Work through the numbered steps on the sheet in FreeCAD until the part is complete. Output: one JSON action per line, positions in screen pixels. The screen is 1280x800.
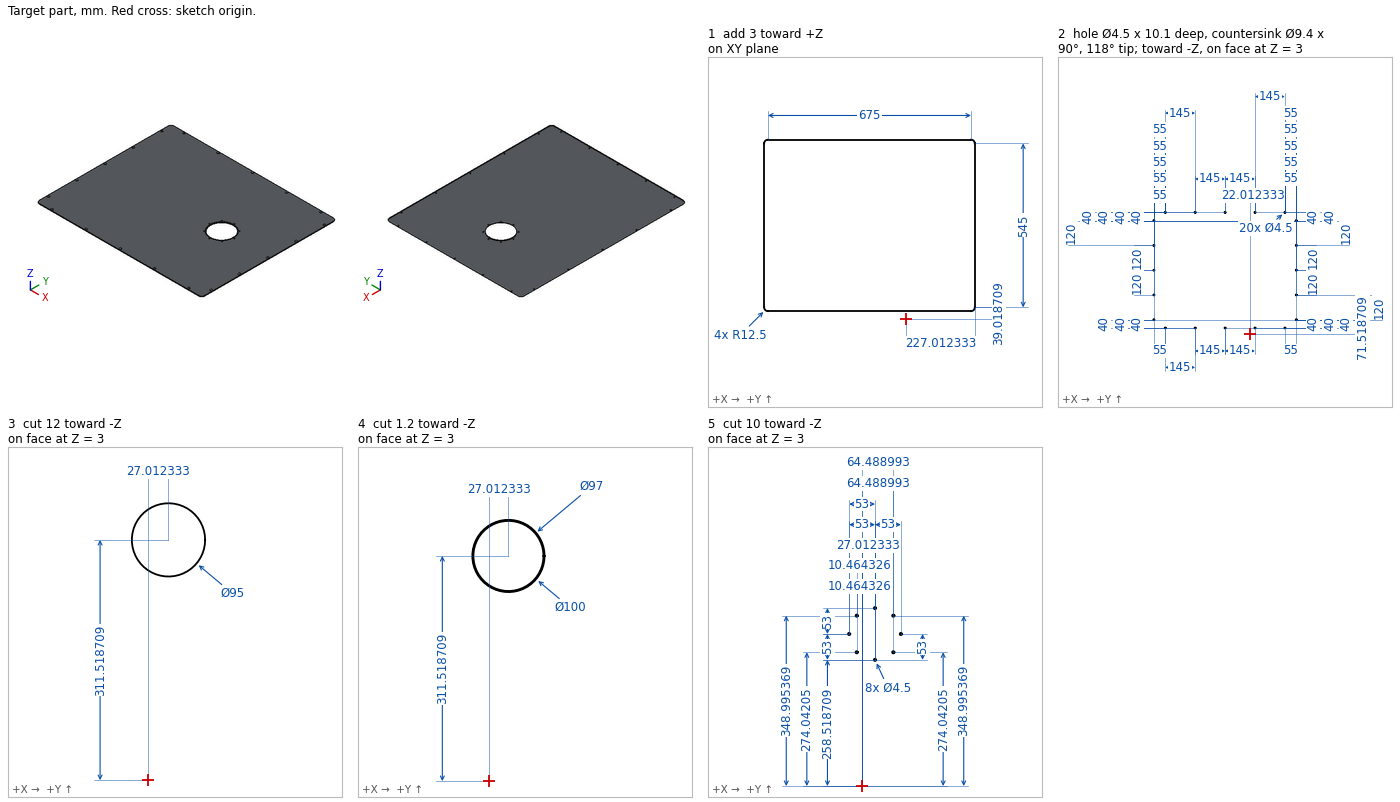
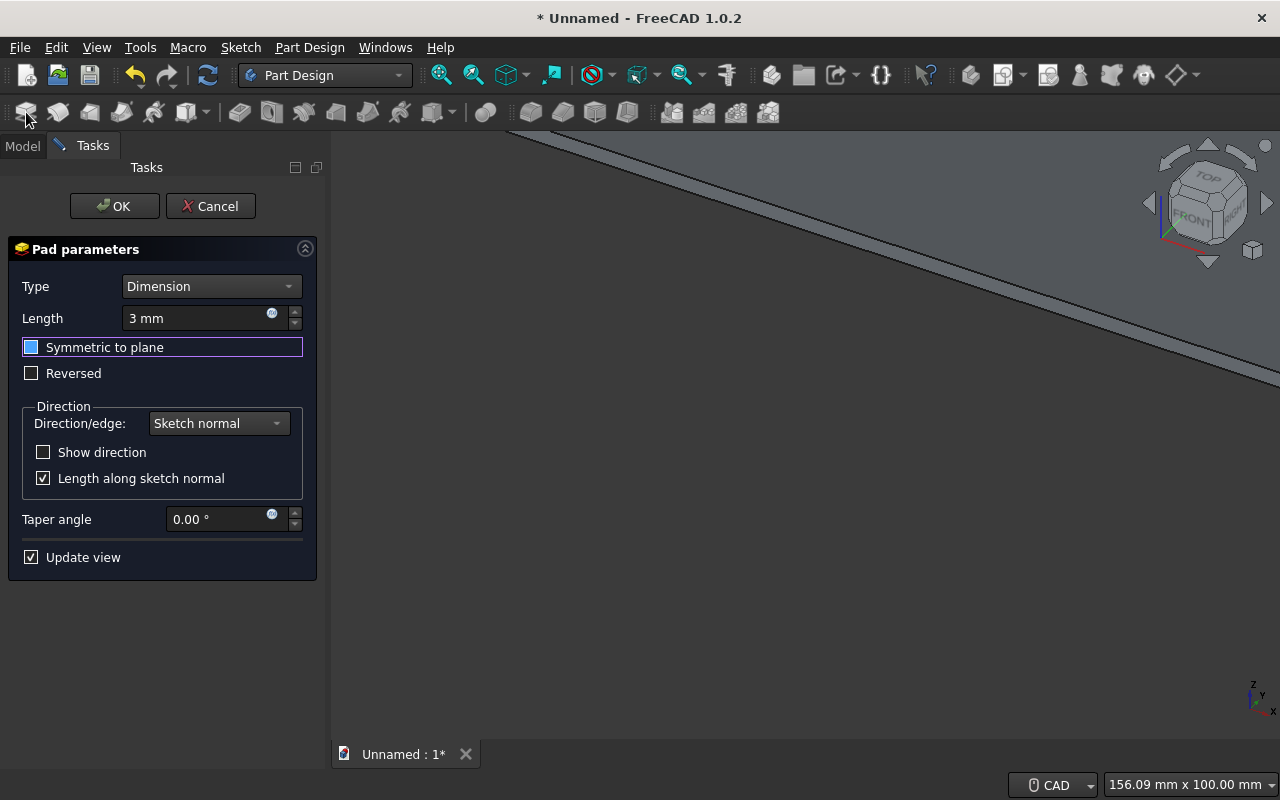
{"action": "left_click", "coordinate": [115, 206]}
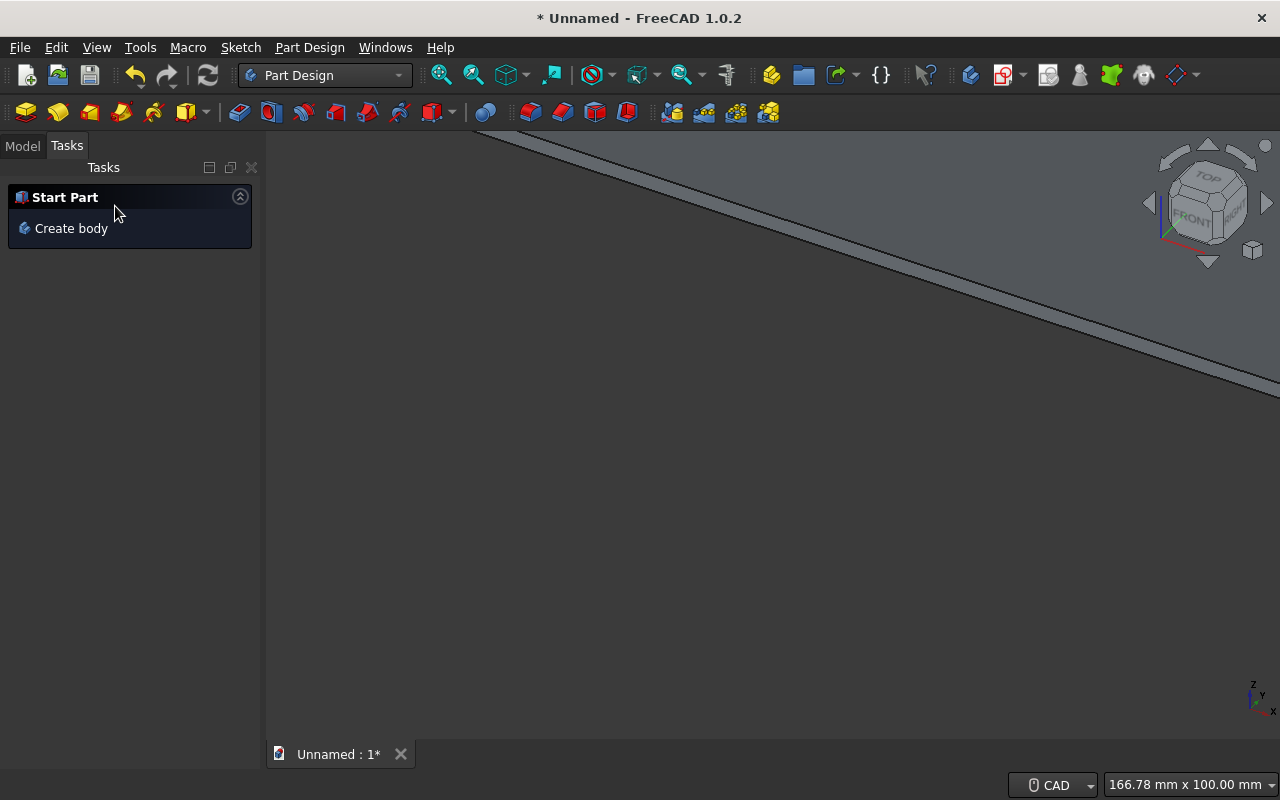
{"action": "left_click", "coordinate": [442, 76]}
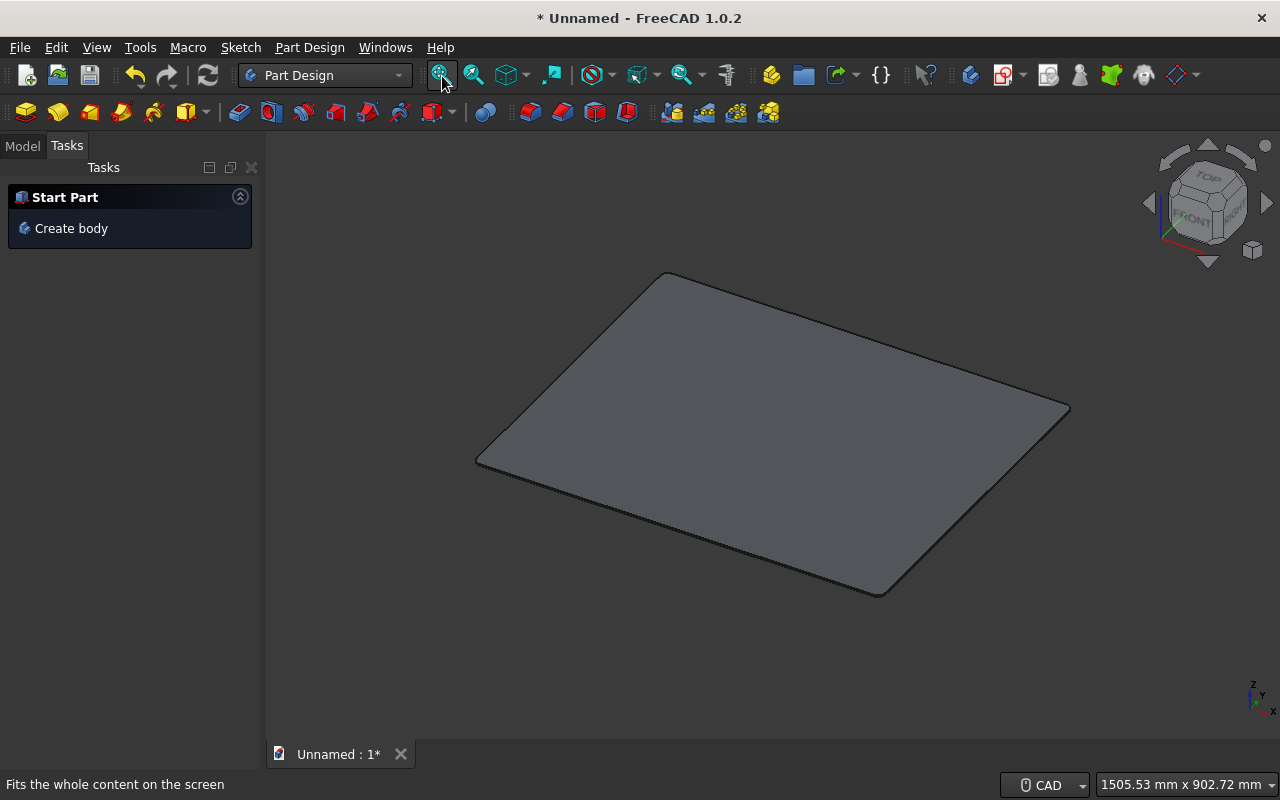
{"action": "left_click", "coordinate": [773, 433]}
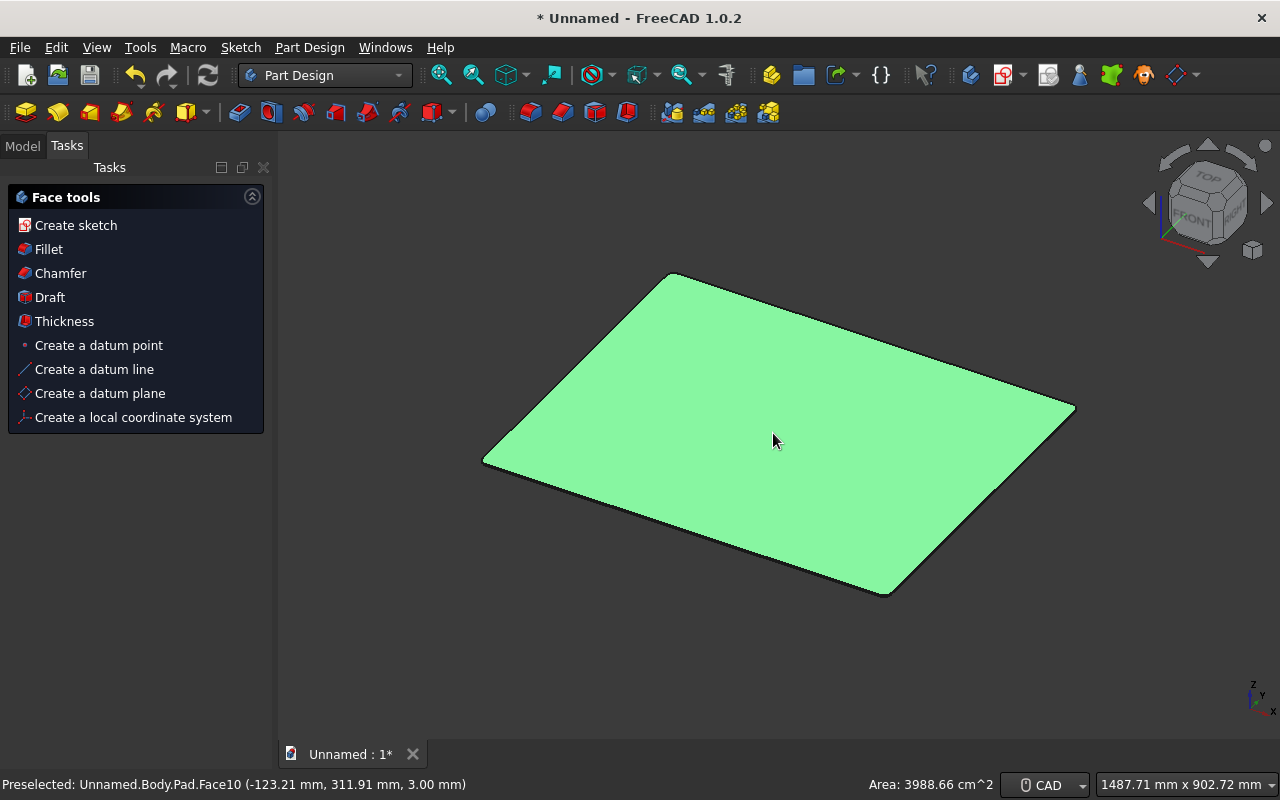
{"action": "left_click", "coordinate": [1004, 76]}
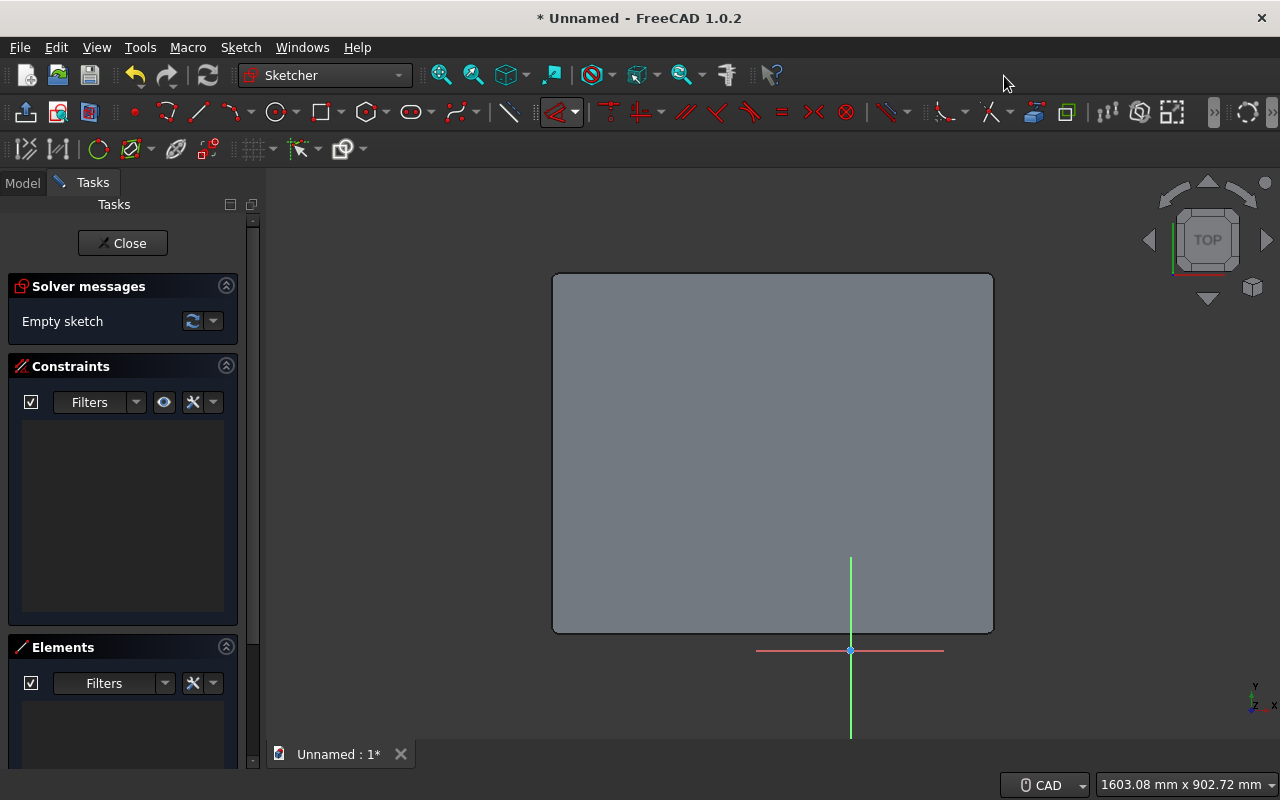
{"action": "left_click", "coordinate": [276, 112]}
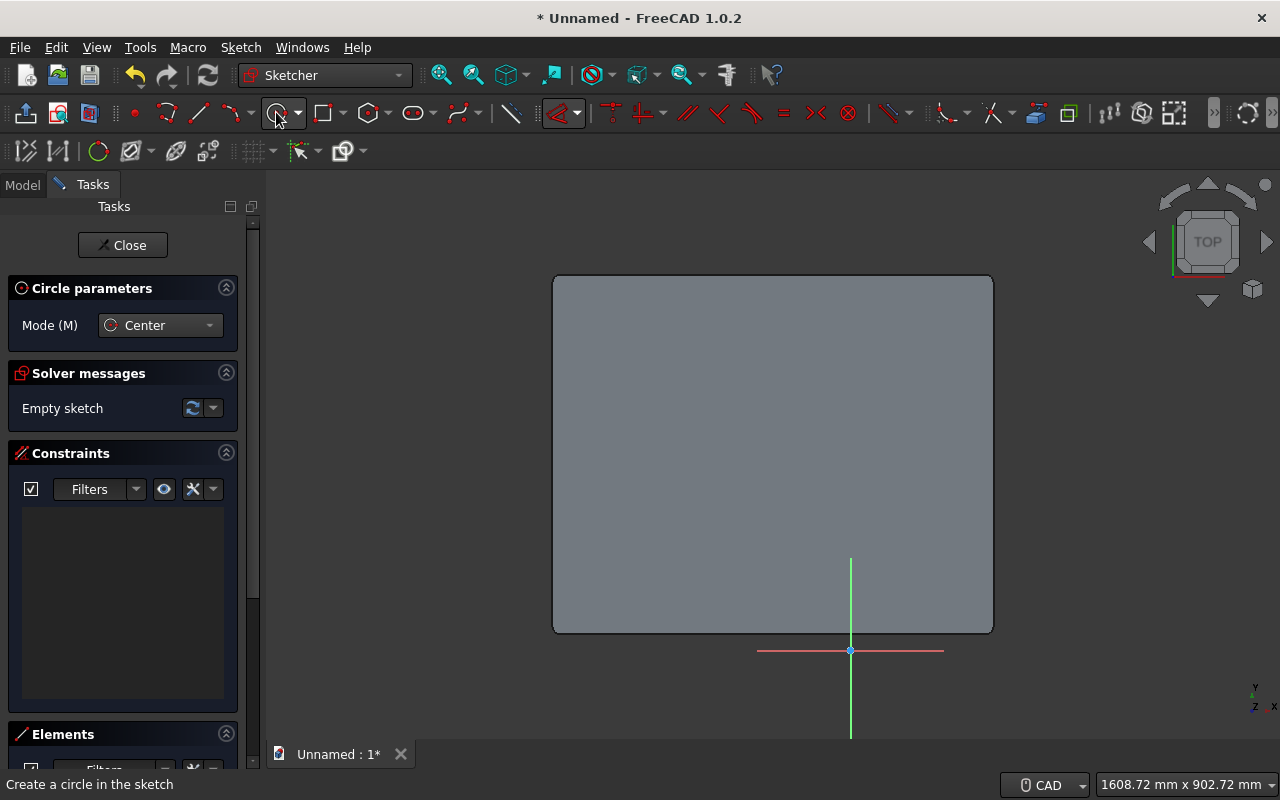
{"action": "scroll", "coordinate": [990, 606], "scroll_direction": "up", "scroll_amount": 14}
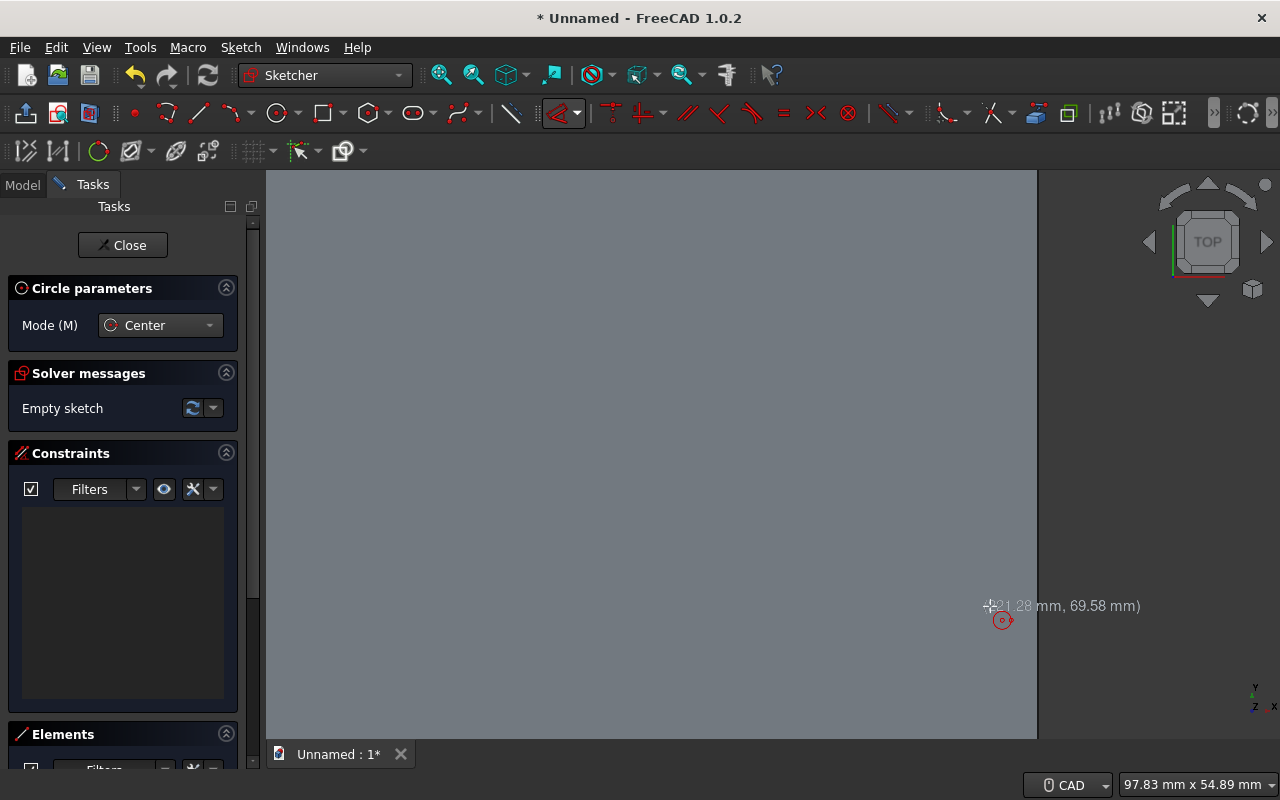
{"action": "scroll", "coordinate": [918, 597], "scroll_direction": "down", "scroll_amount": 14}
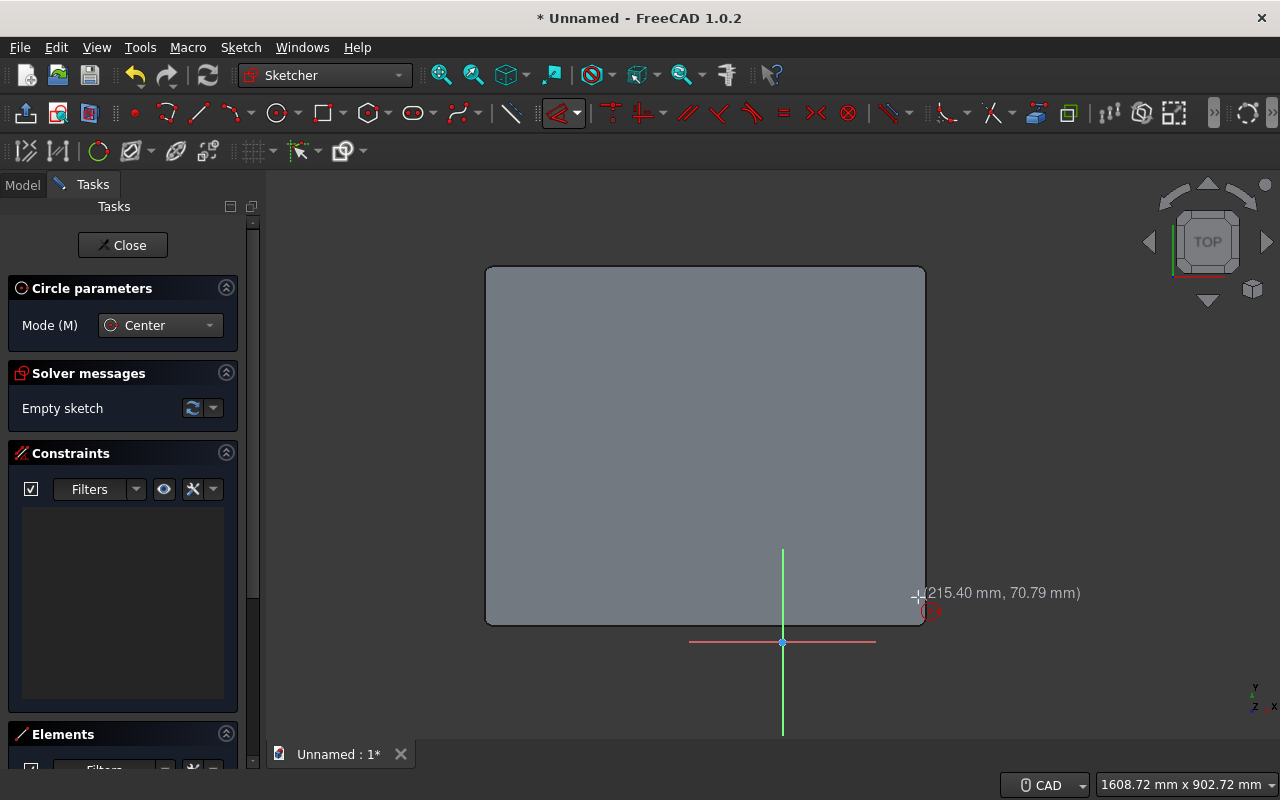
{"action": "left_click", "coordinate": [923, 597]}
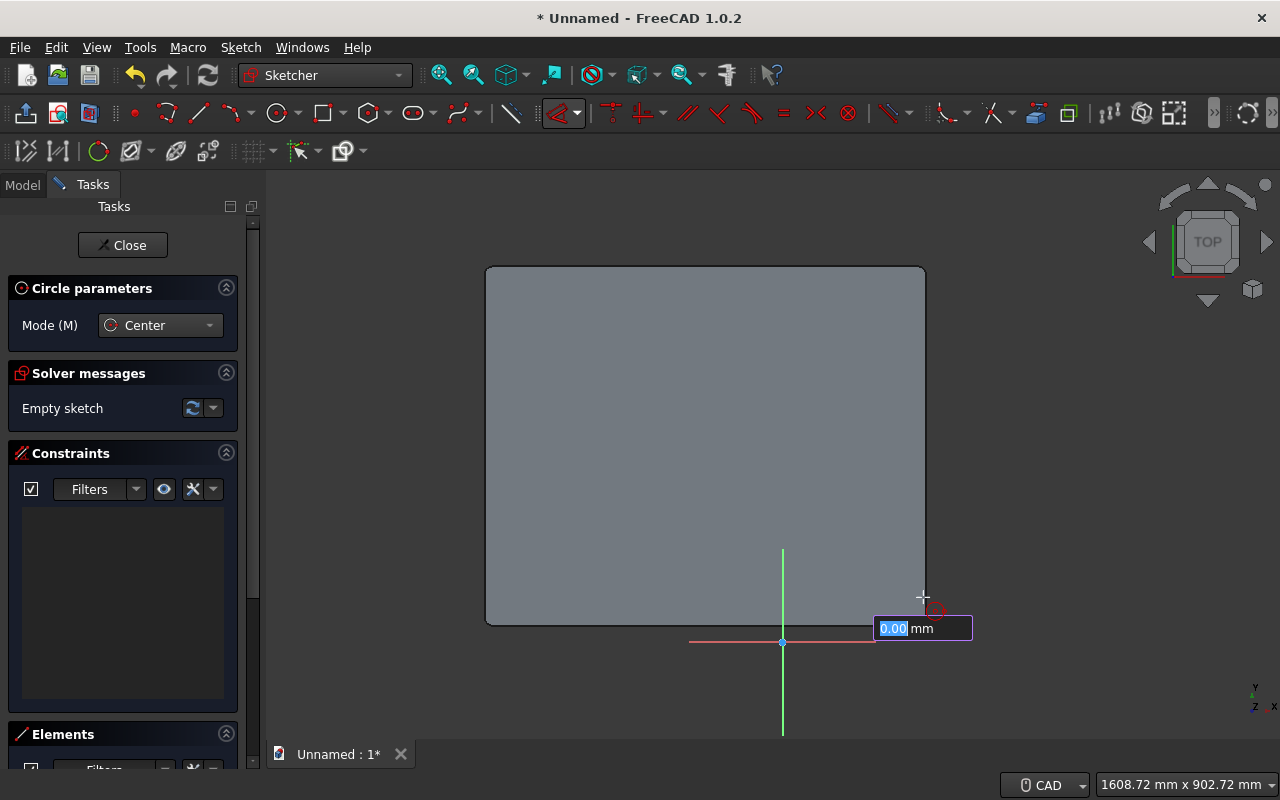
{"action": "scroll", "coordinate": [924, 596], "scroll_direction": "up", "scroll_amount": 13}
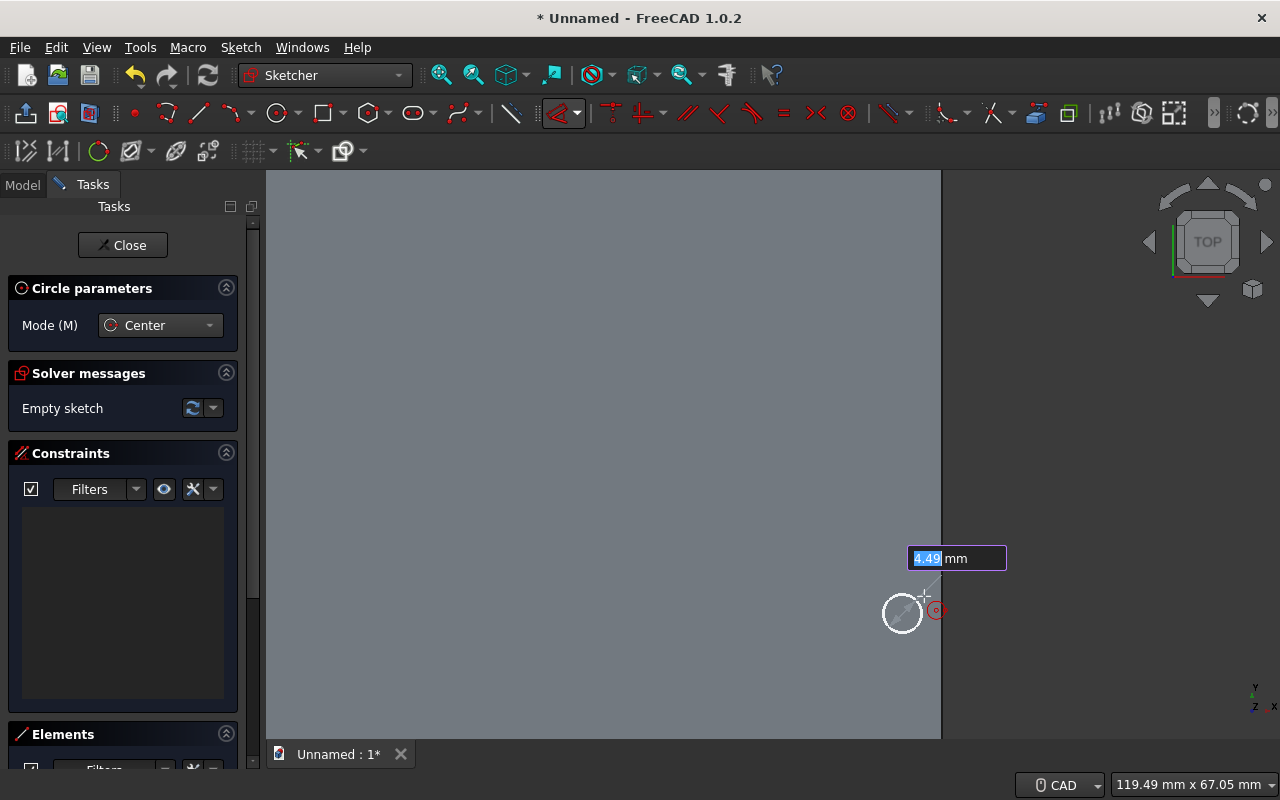
{"action": "left_click", "coordinate": [913, 591]}